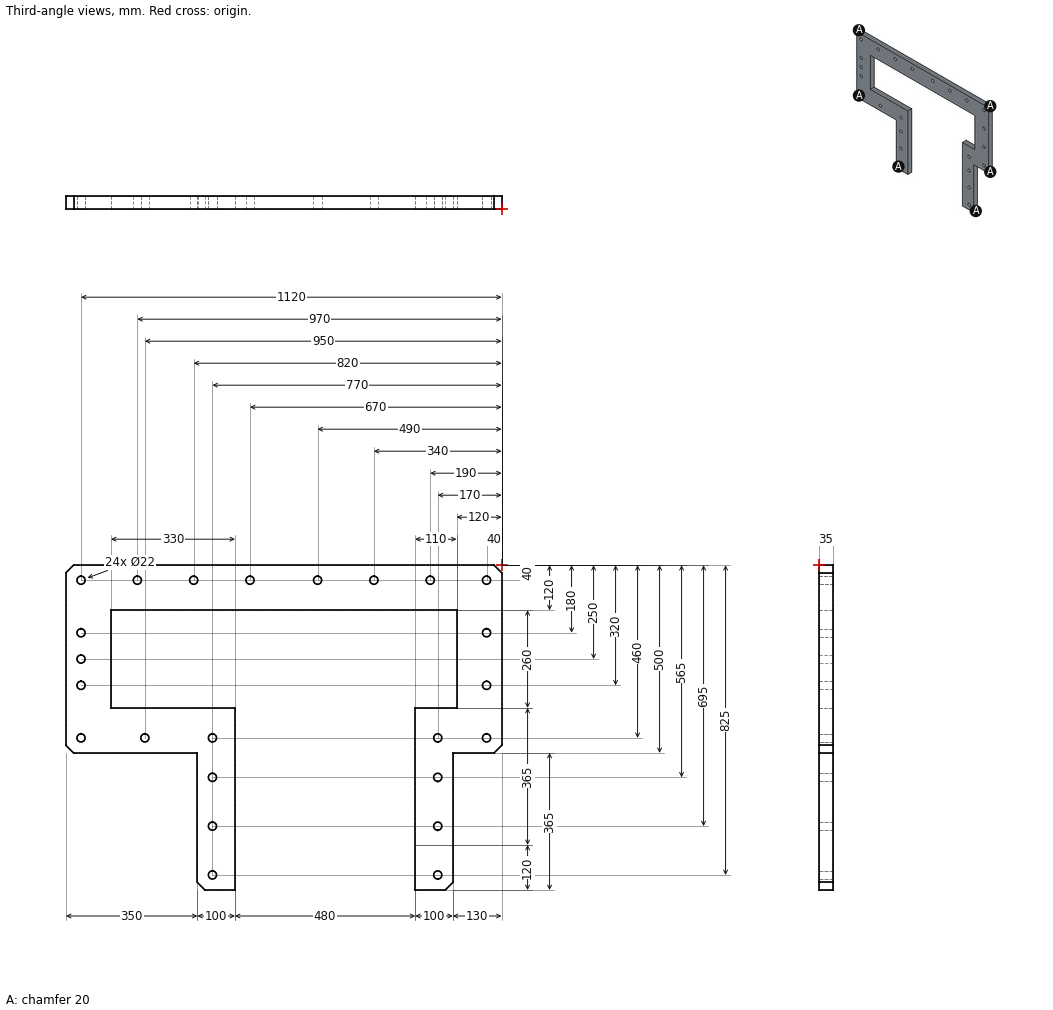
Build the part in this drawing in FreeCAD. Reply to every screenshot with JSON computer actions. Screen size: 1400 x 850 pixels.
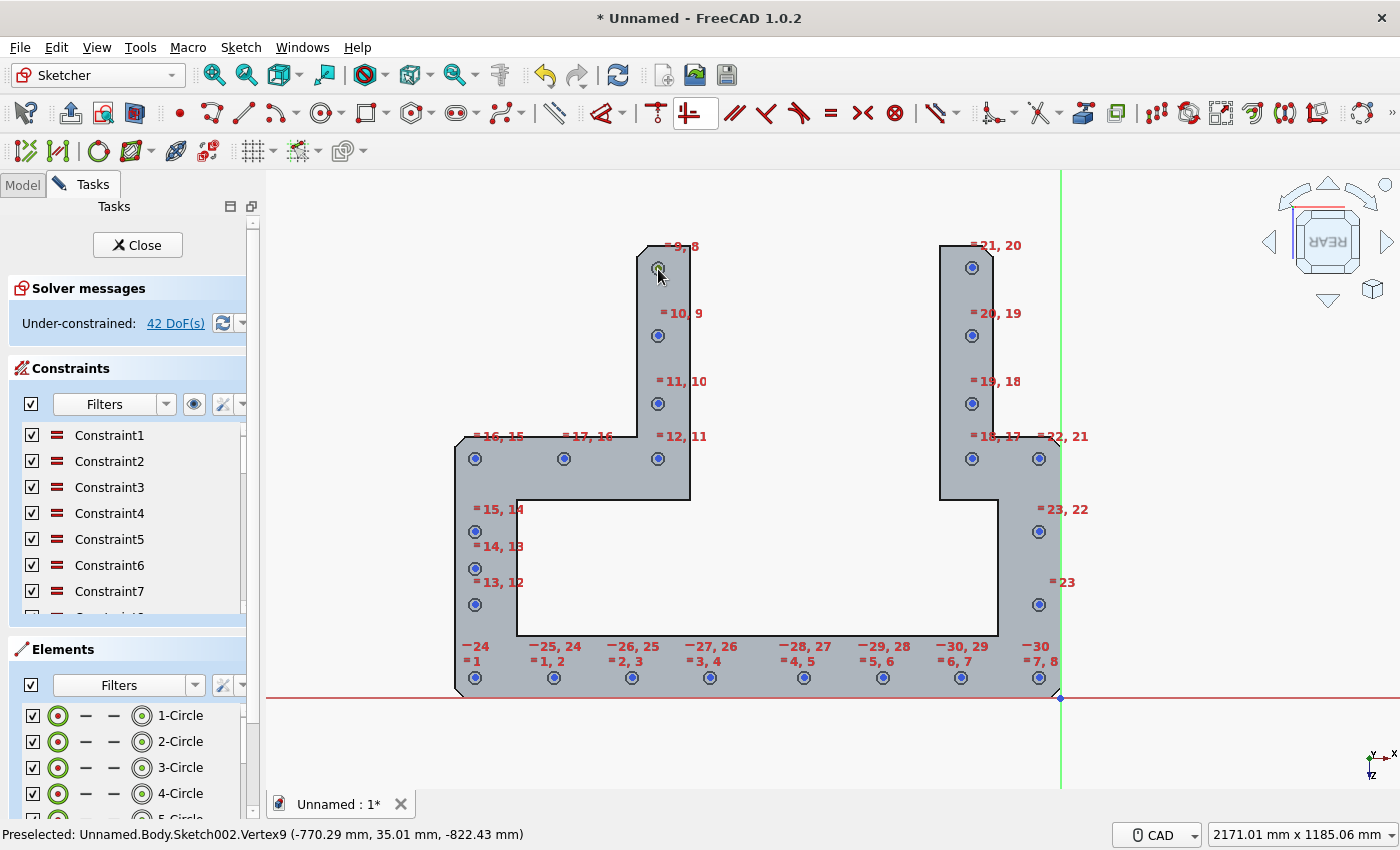
{"action": "left_click", "coordinate": [658, 336]}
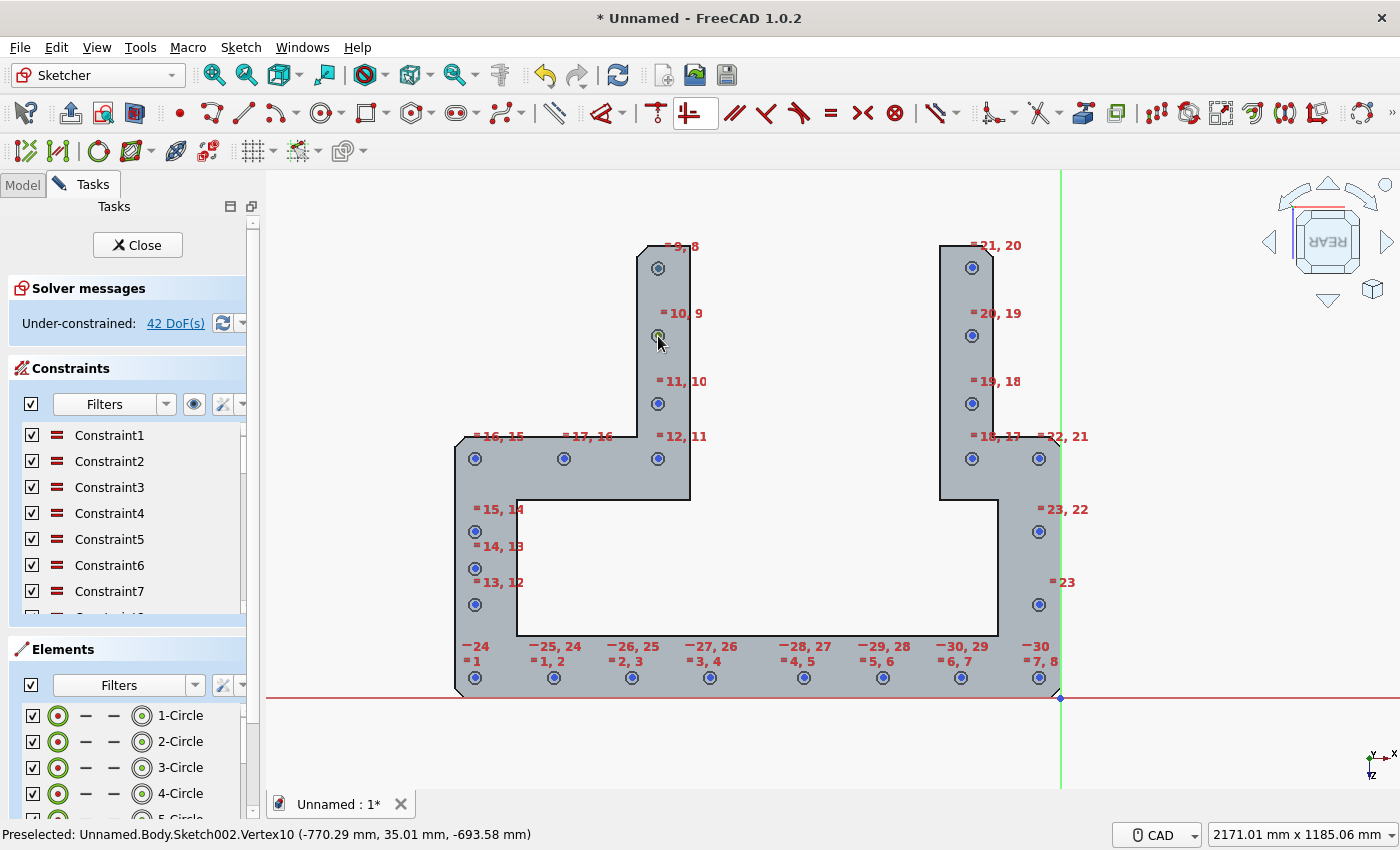
{"action": "left_click", "coordinate": [712, 114]}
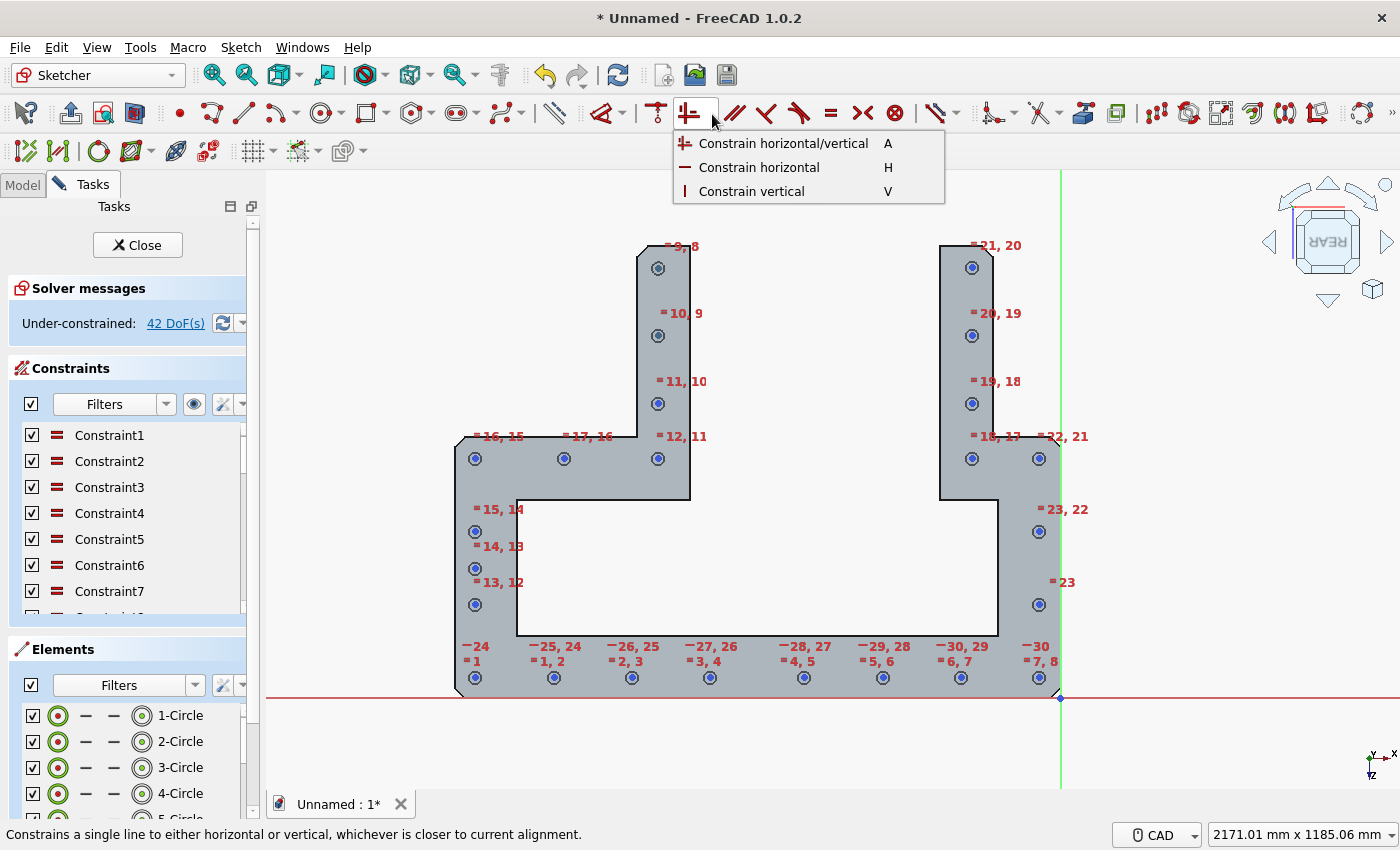
{"action": "left_click", "coordinate": [809, 191]}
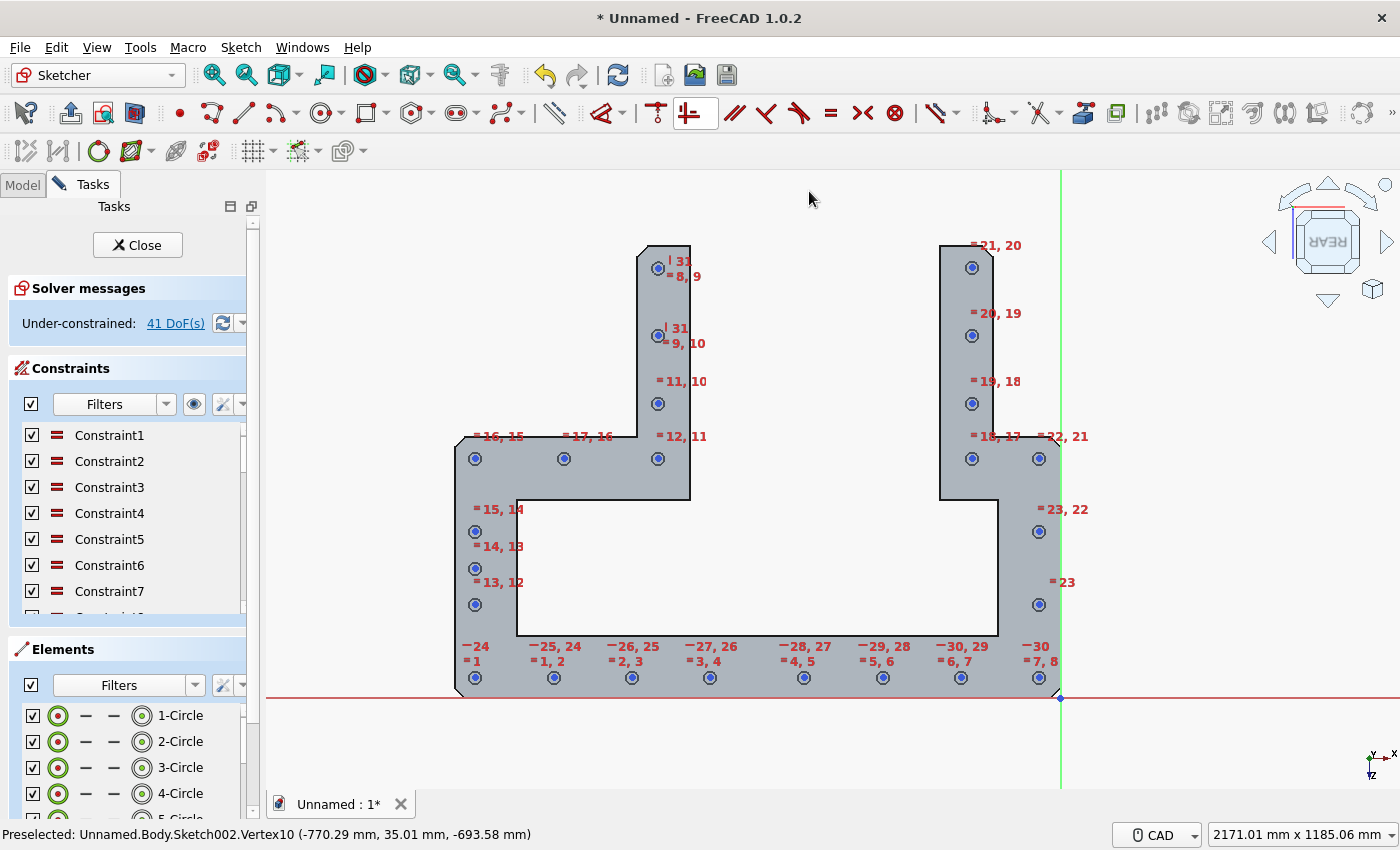
{"action": "left_click", "coordinate": [658, 336]}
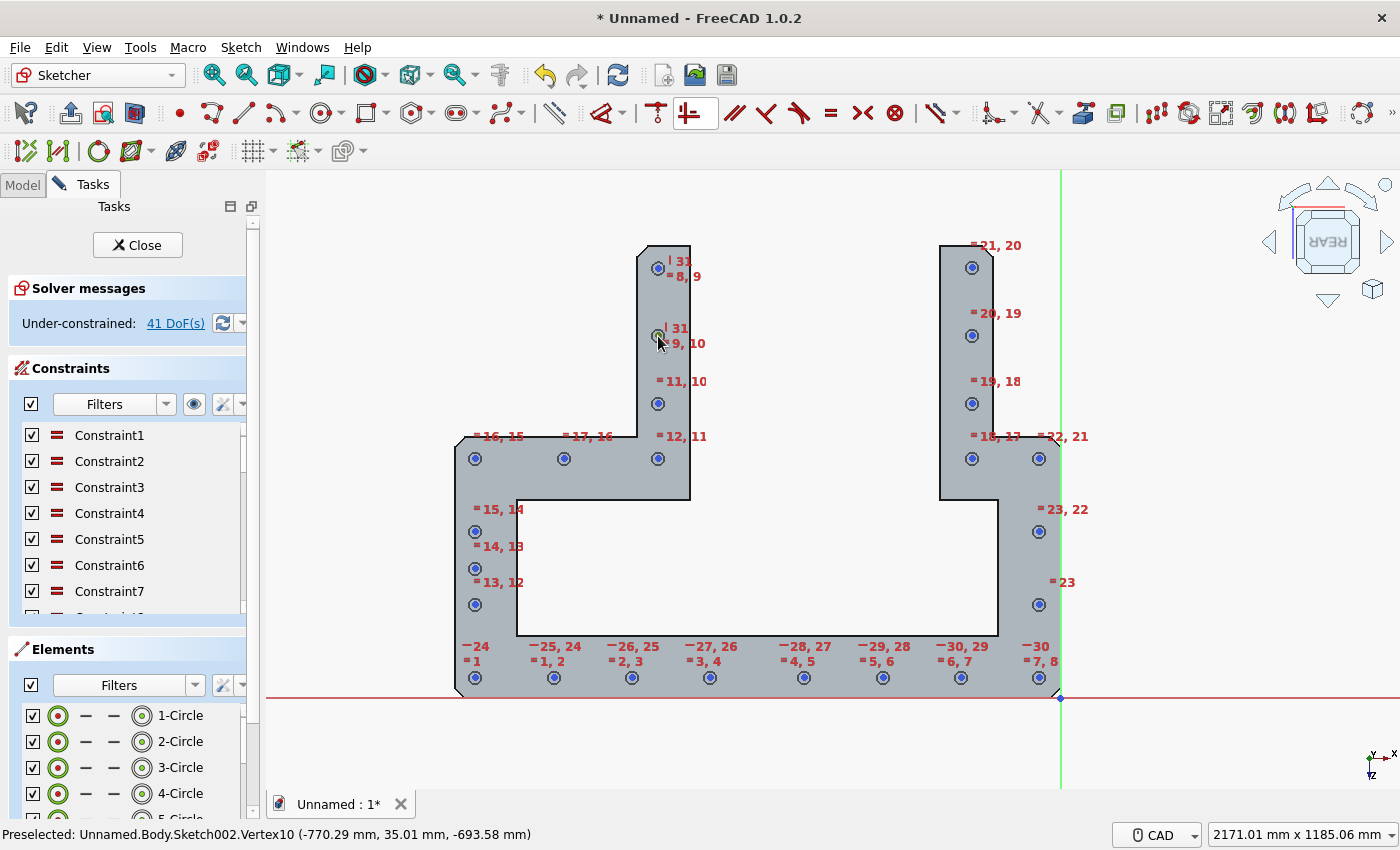
{"action": "left_click", "coordinate": [658, 404]}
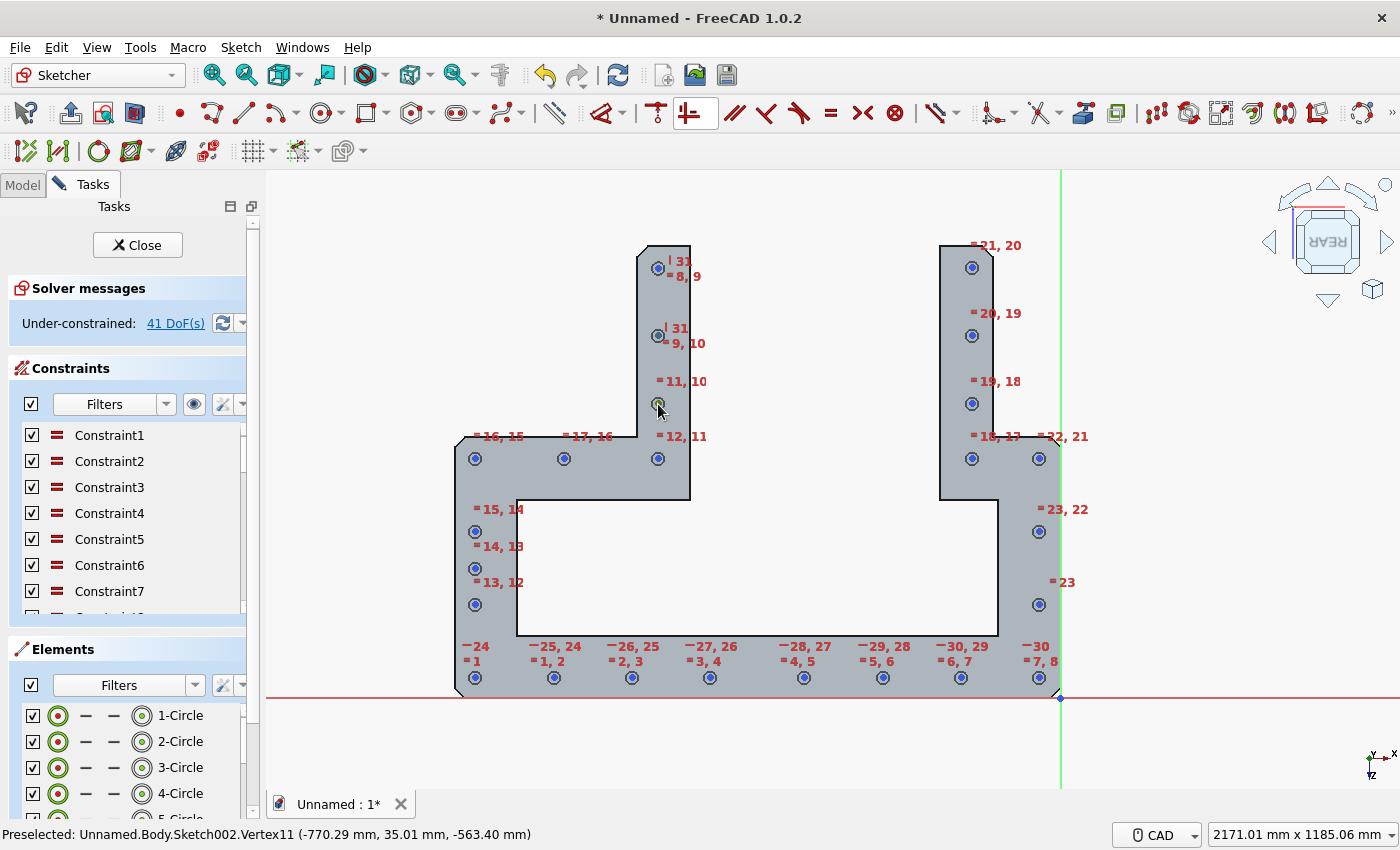
{"action": "key", "text": "v"}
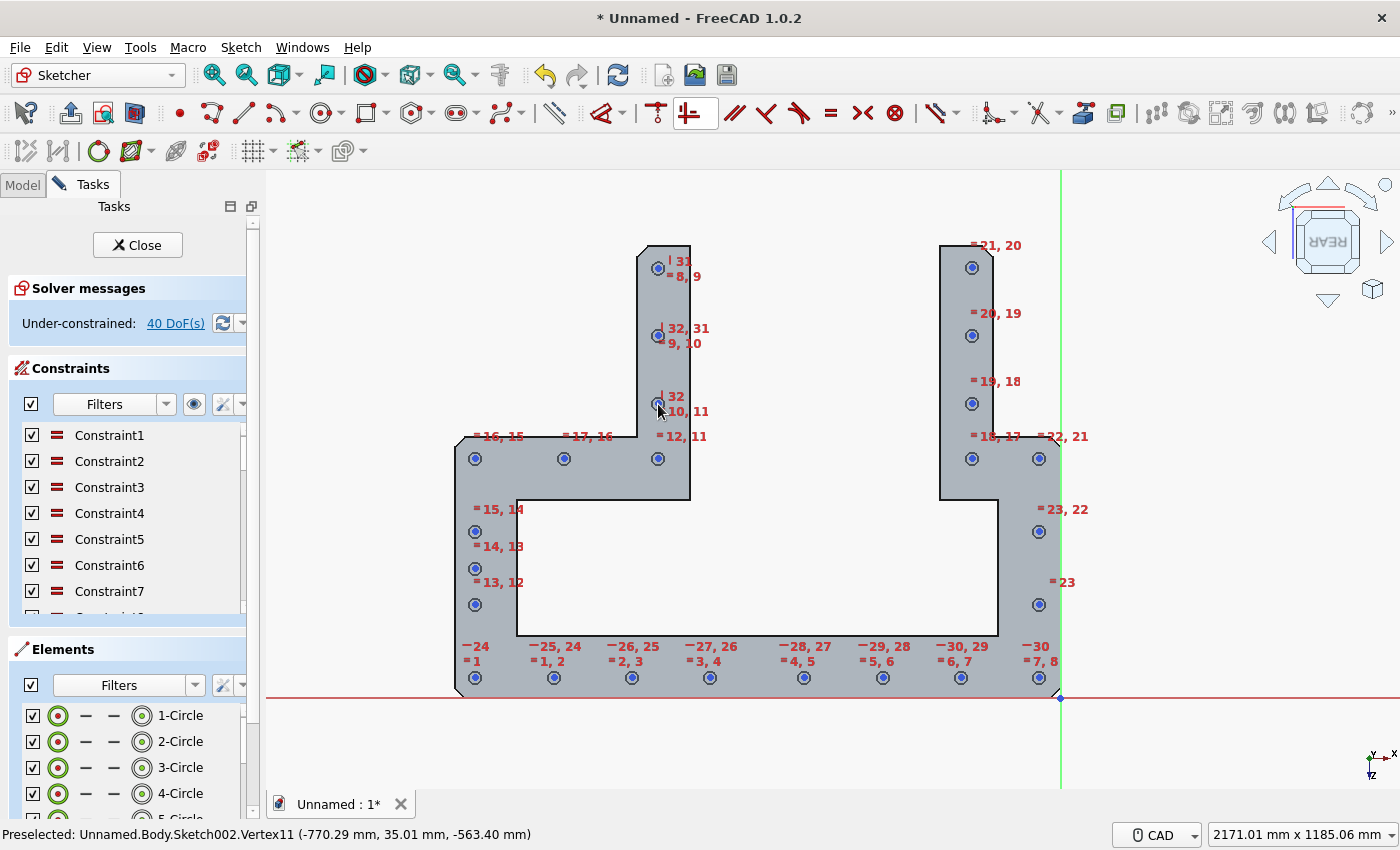
{"action": "left_click", "coordinate": [656, 406]}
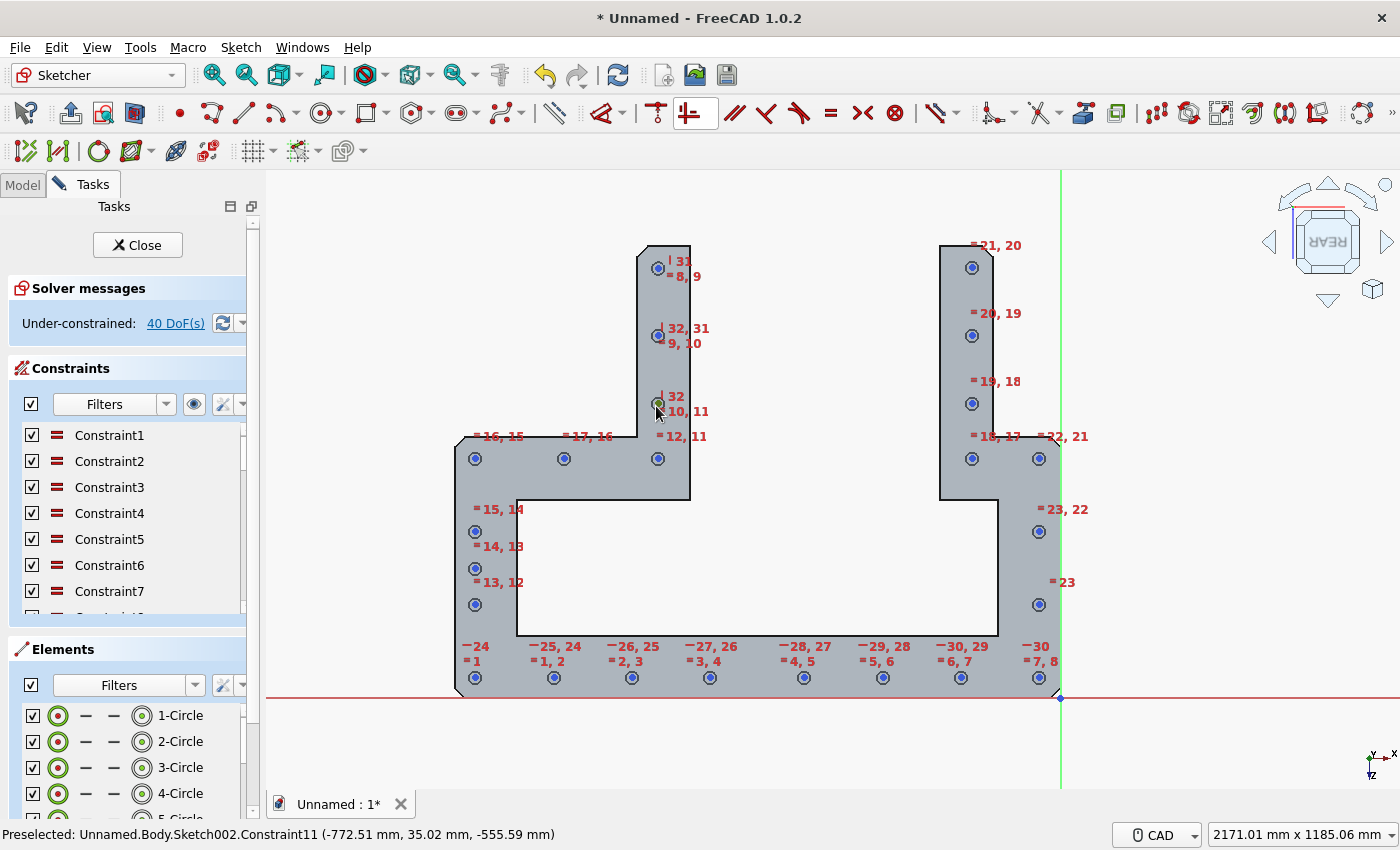
{"action": "left_click", "coordinate": [658, 459]}